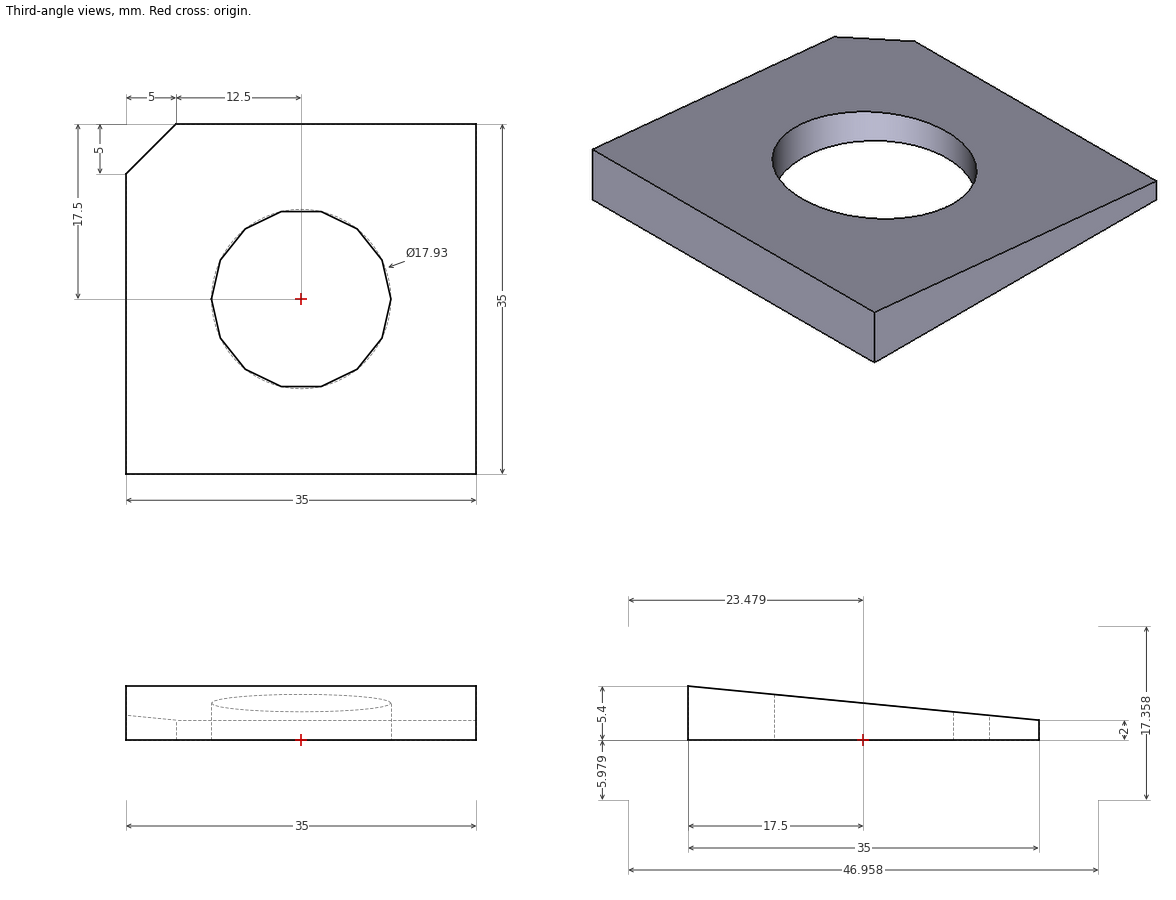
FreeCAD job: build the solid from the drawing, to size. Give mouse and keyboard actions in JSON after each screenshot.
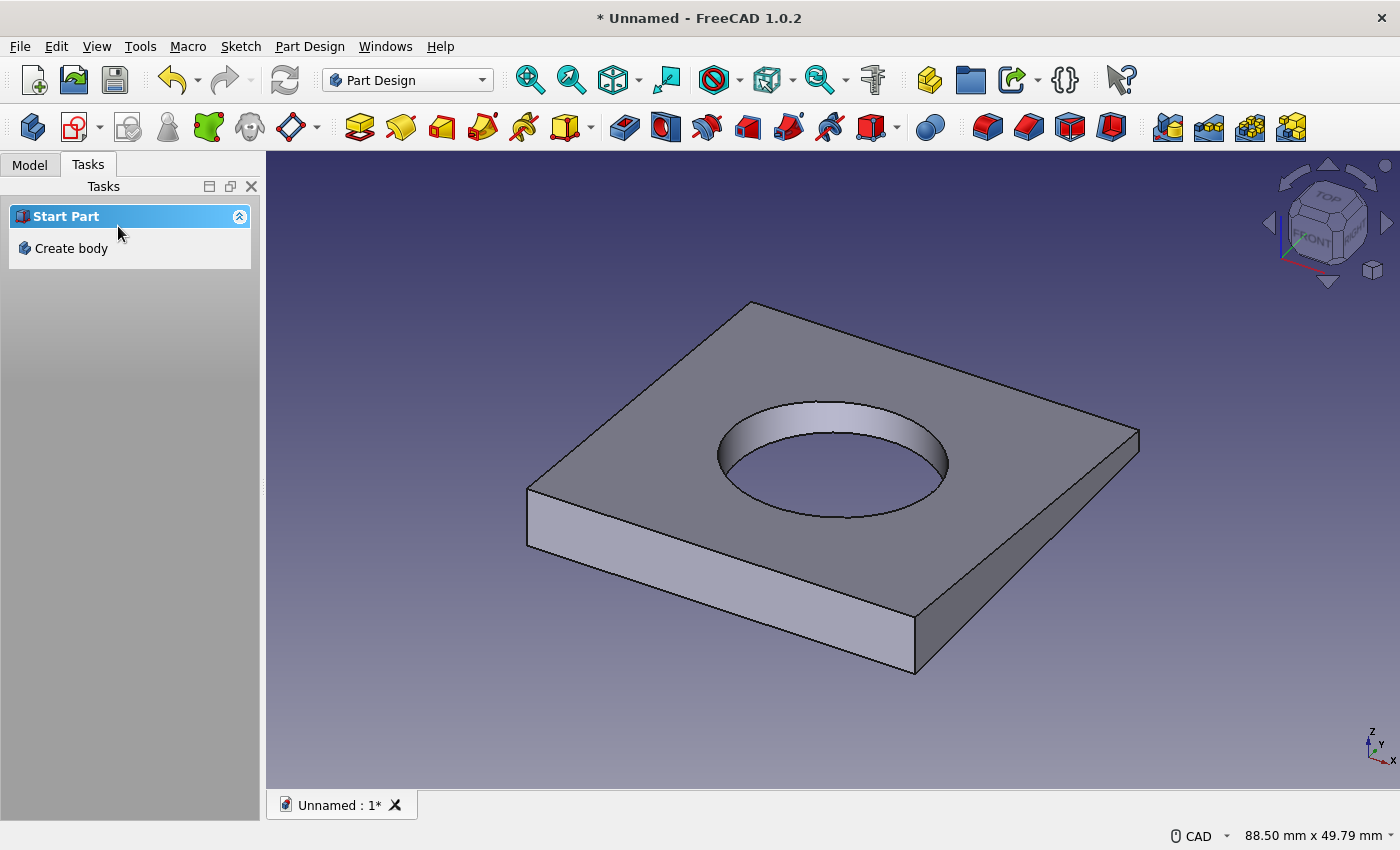
{"action": "key", "text": "5"}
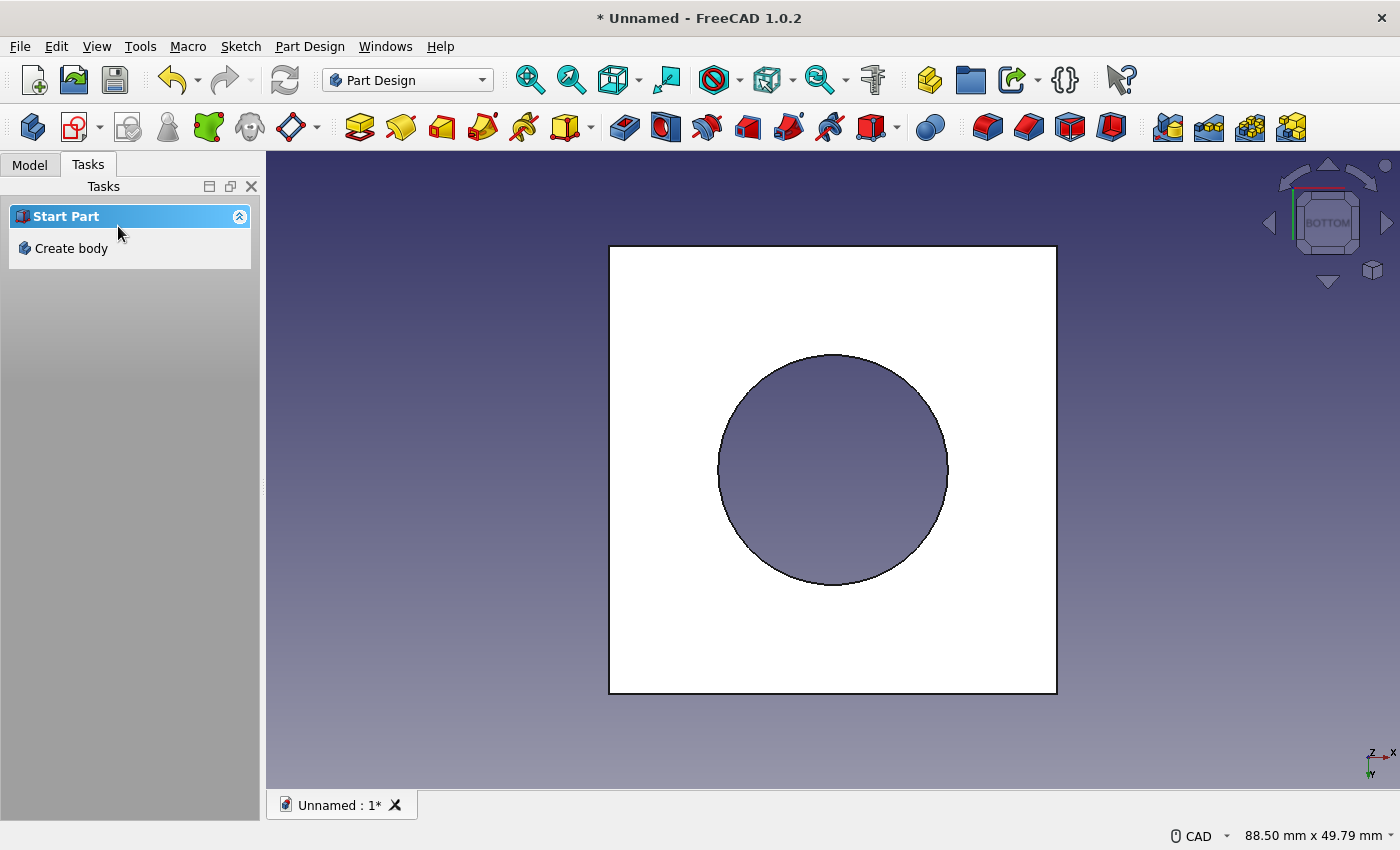
{"action": "left_click", "coordinate": [961, 597]}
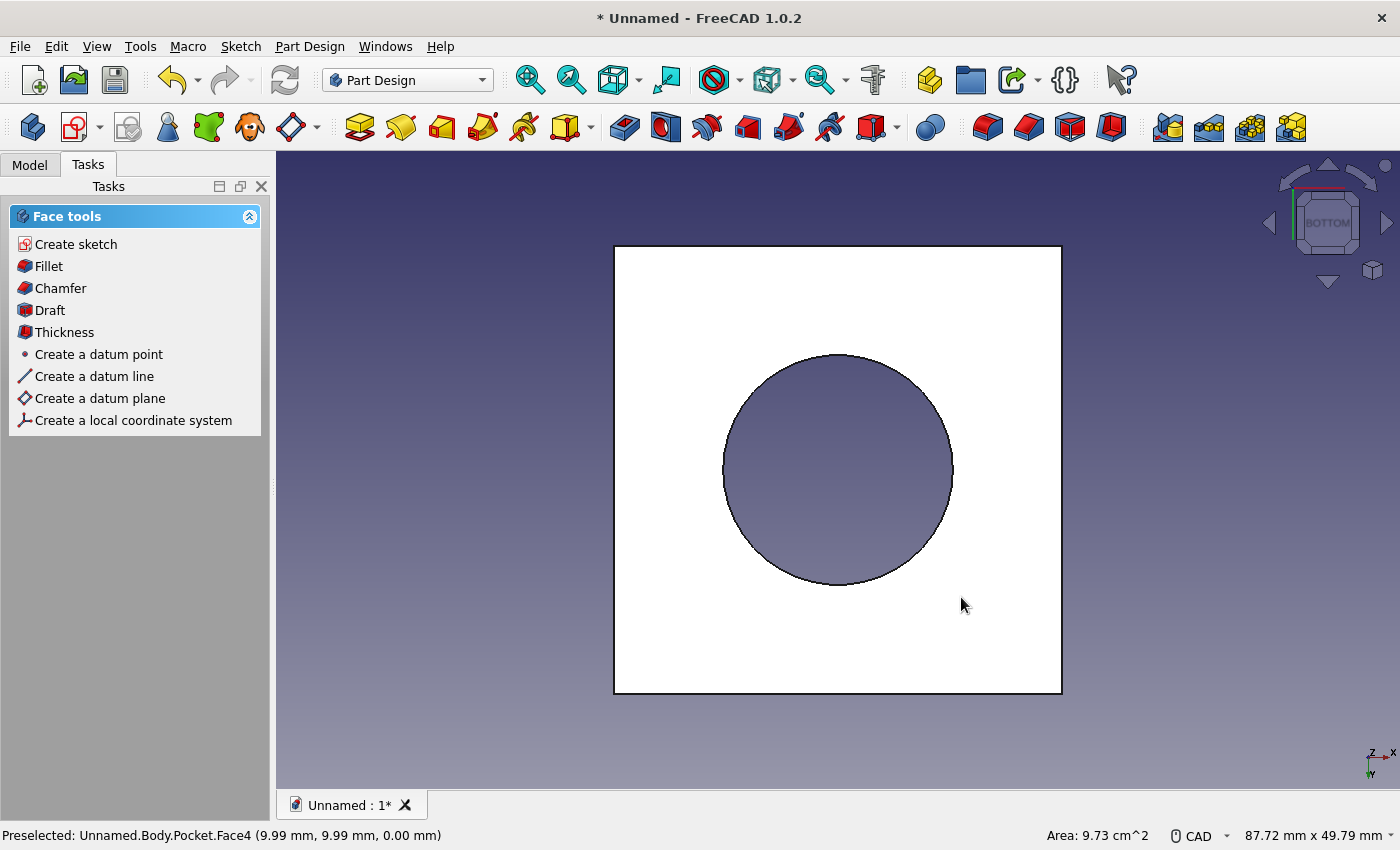
{"action": "left_click", "coordinate": [74, 128]}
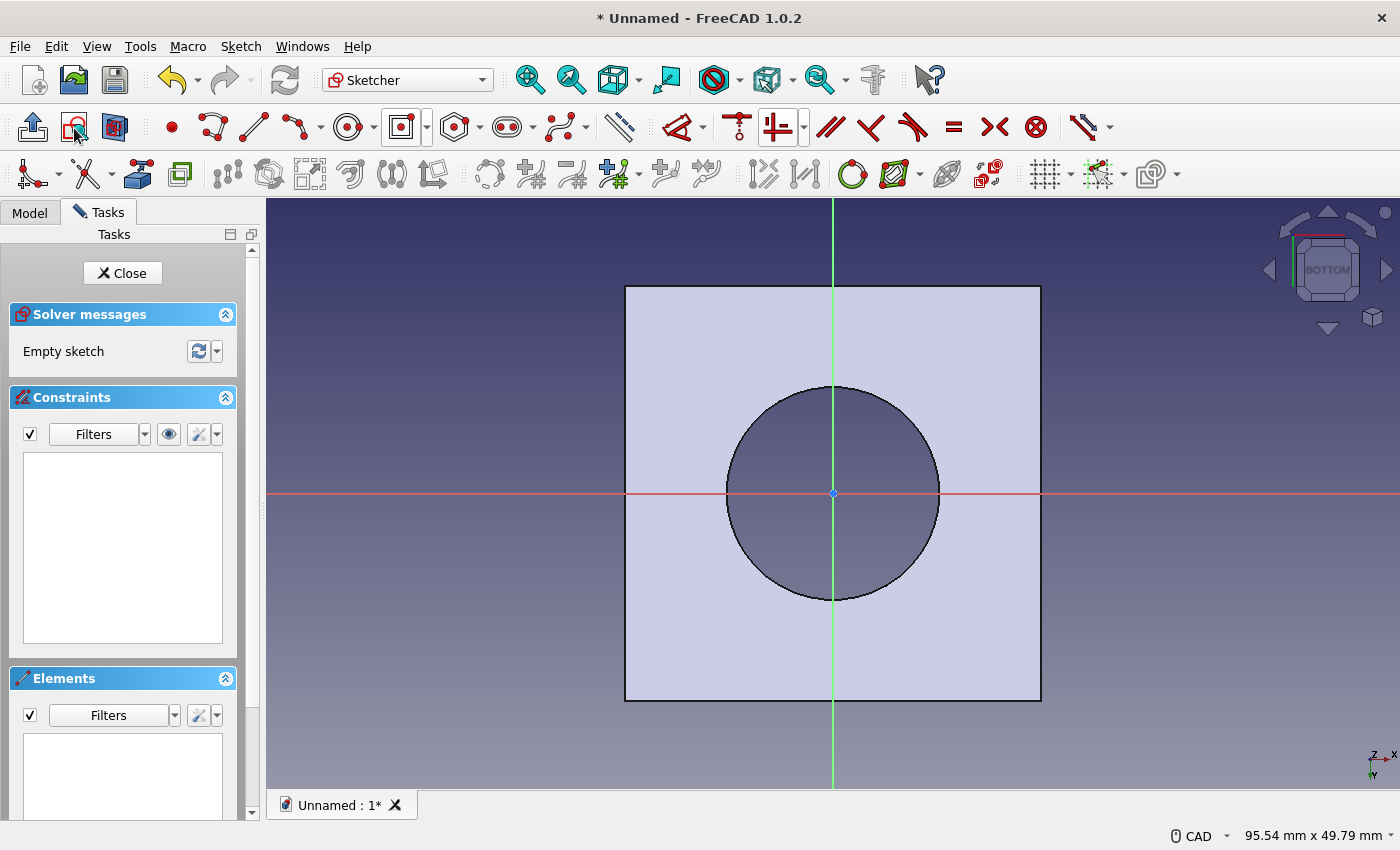
{"action": "scroll", "coordinate": [633, 707], "scroll_direction": "up", "scroll_amount": 9}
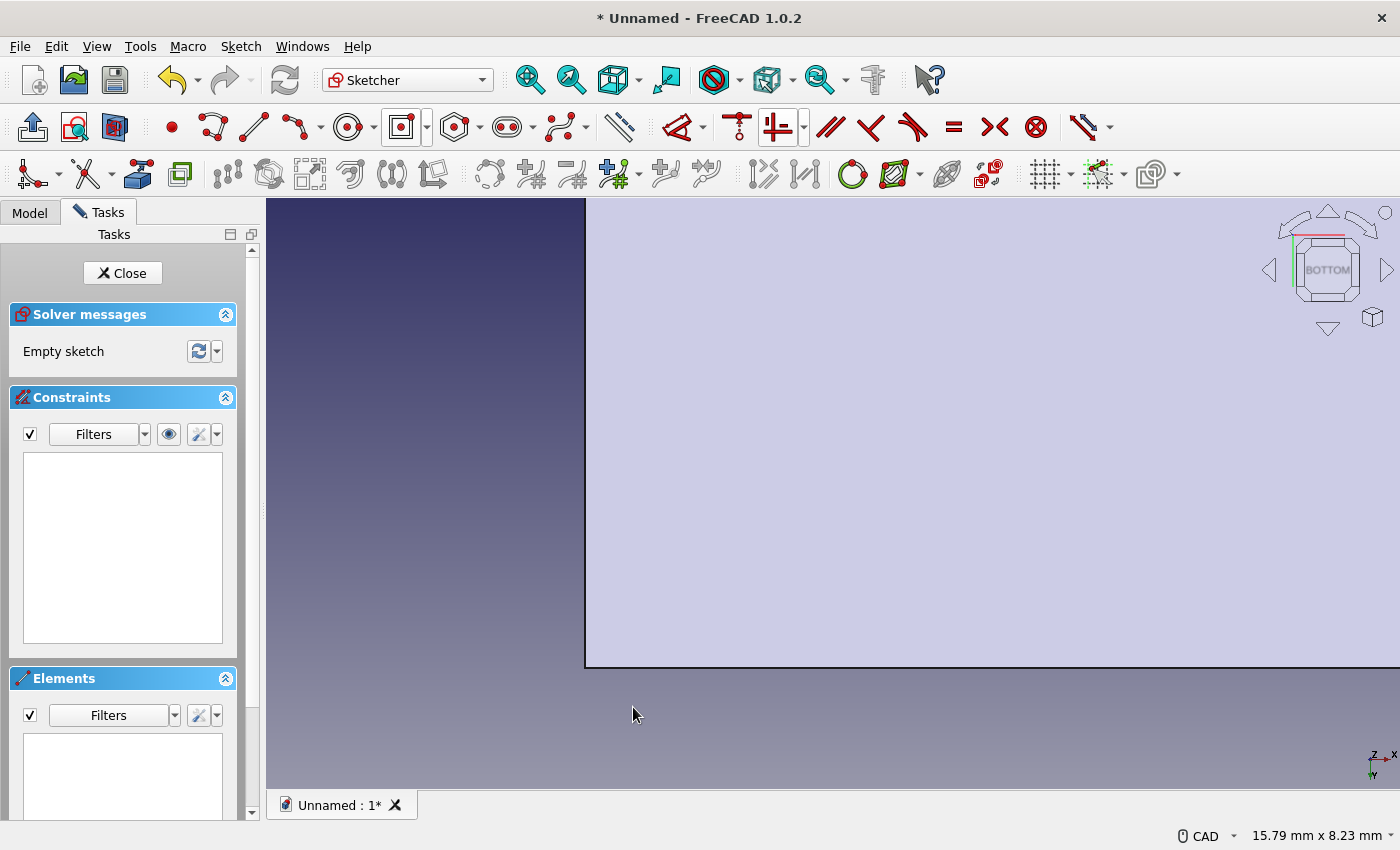
{"action": "key", "text": "g m"}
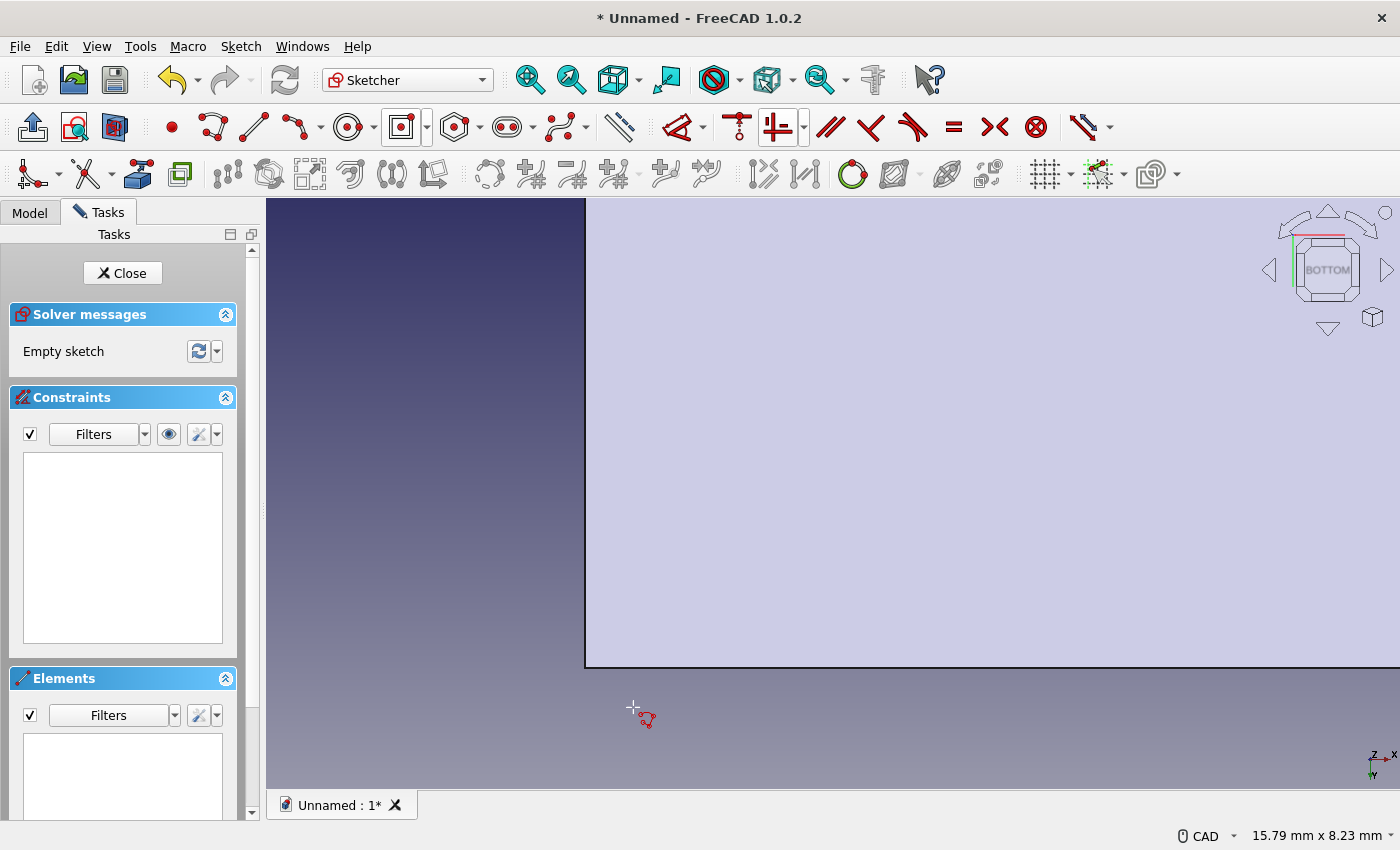
{"action": "left_click", "coordinate": [944, 668]}
{"action": "left_click", "coordinate": [585, 309]}
{"action": "left_click", "coordinate": [585, 668]}
{"action": "left_click", "coordinate": [944, 669]}
{"action": "key", "text": "Escape"}
{"action": "key", "text": "Escape"}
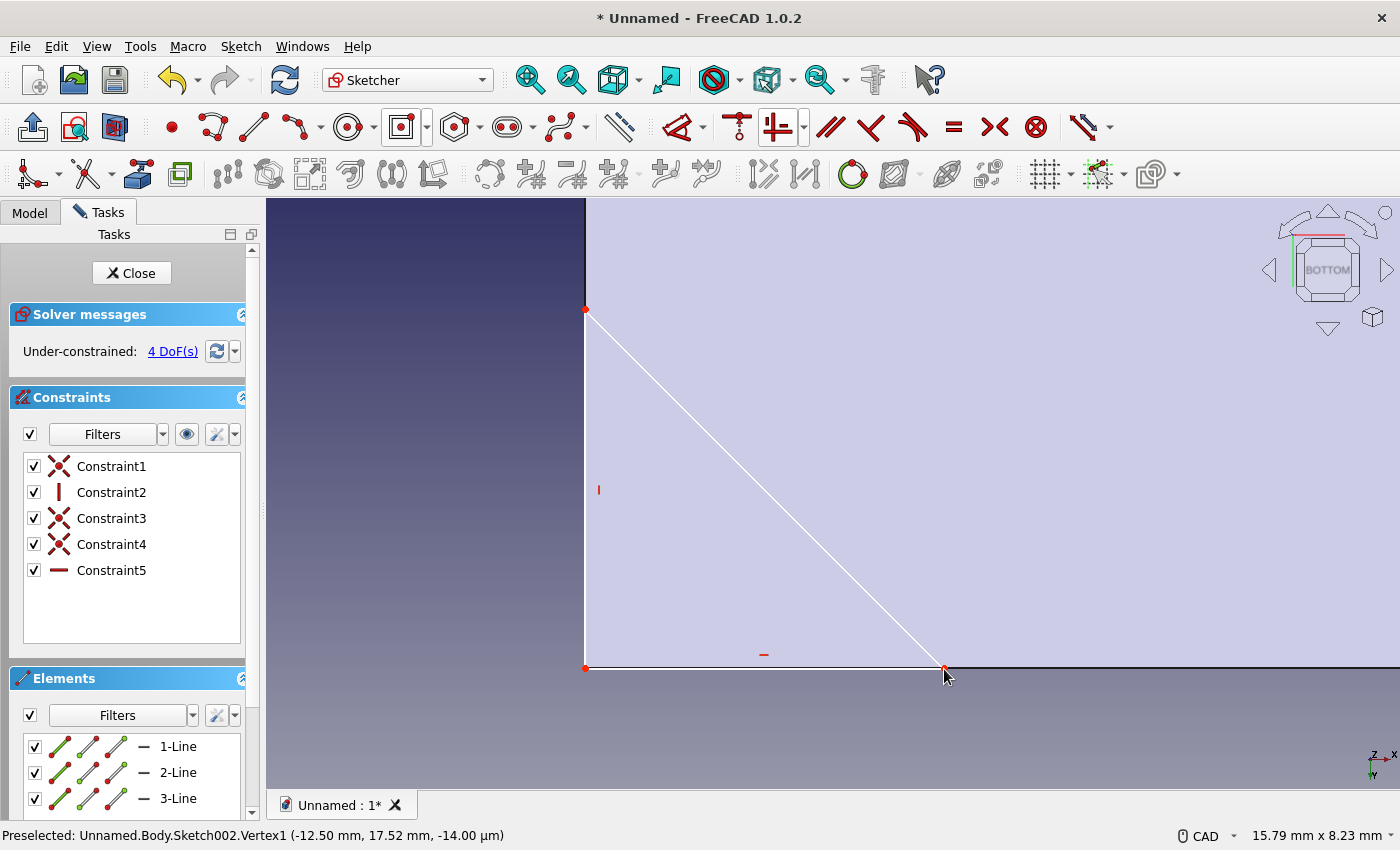
{"action": "left_click", "coordinate": [585, 418]}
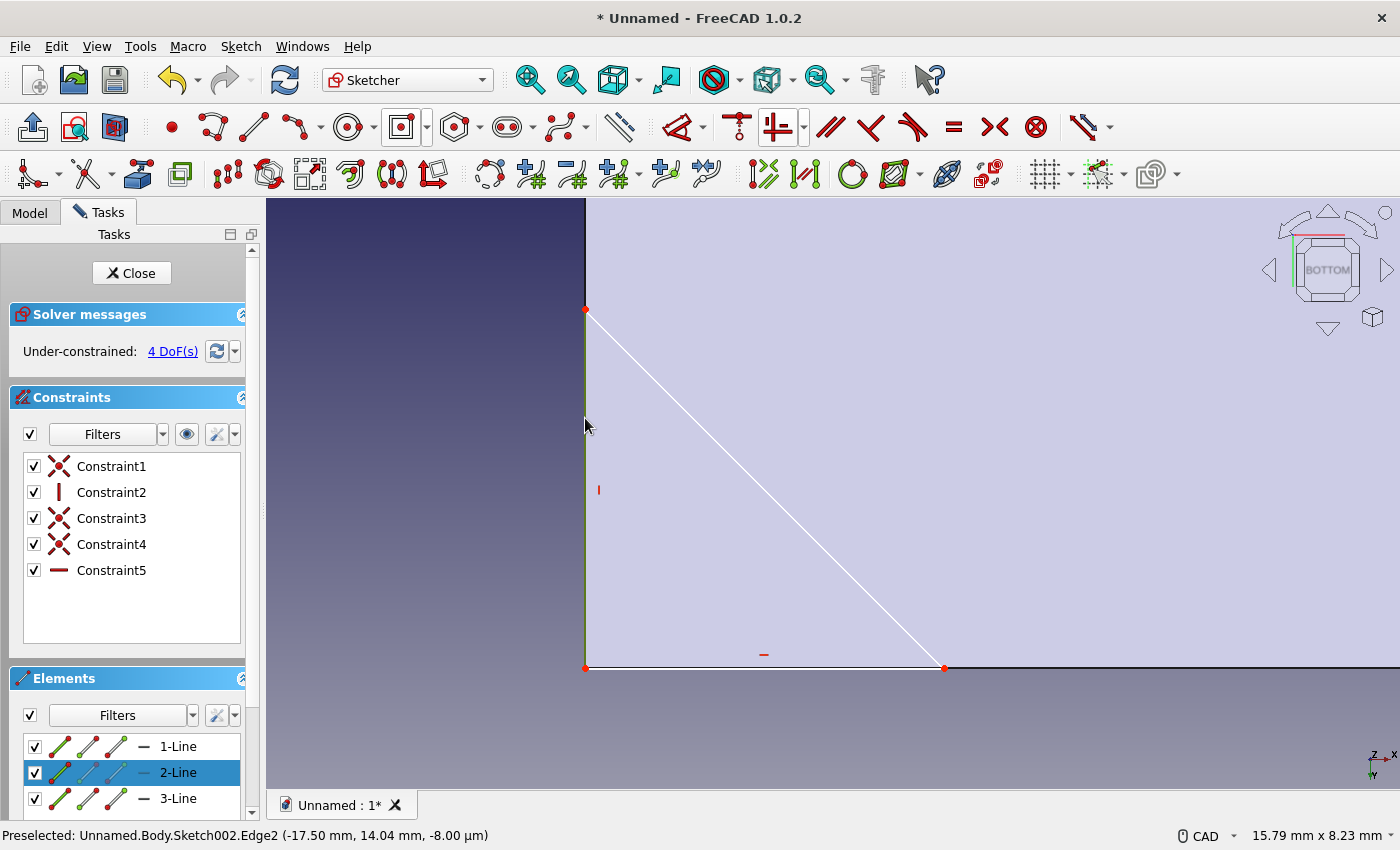
{"action": "key", "text": "i"}